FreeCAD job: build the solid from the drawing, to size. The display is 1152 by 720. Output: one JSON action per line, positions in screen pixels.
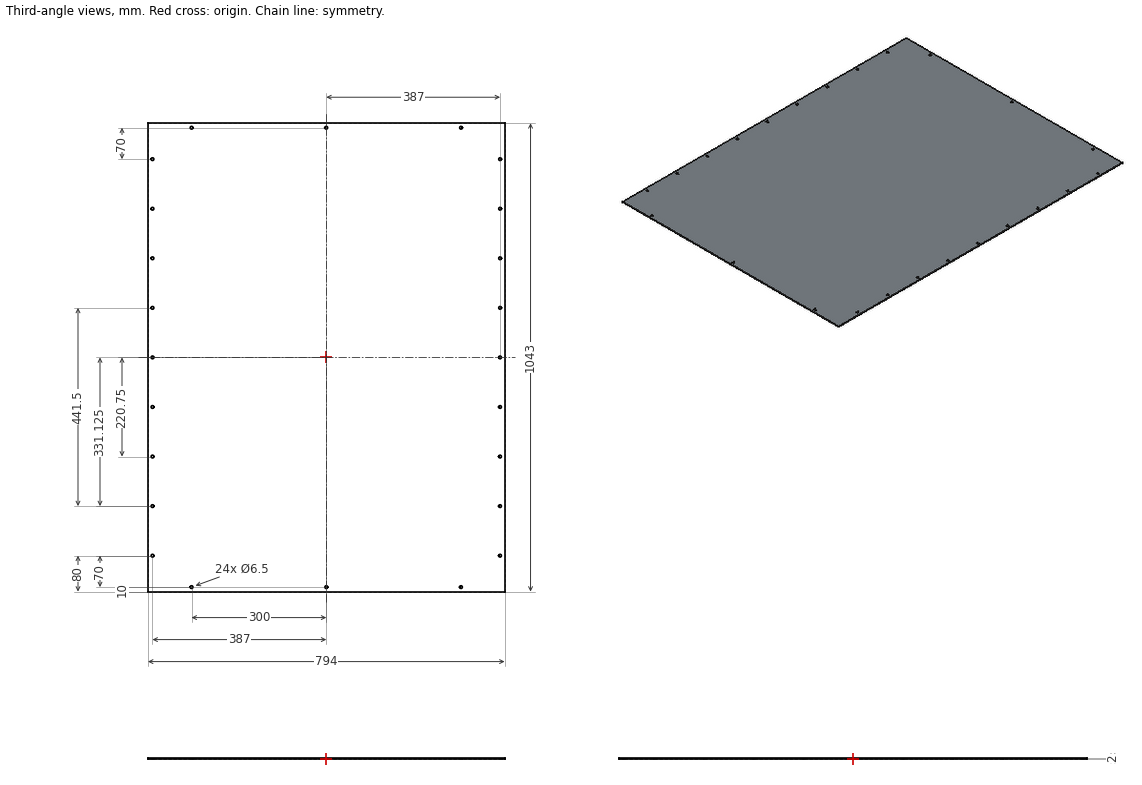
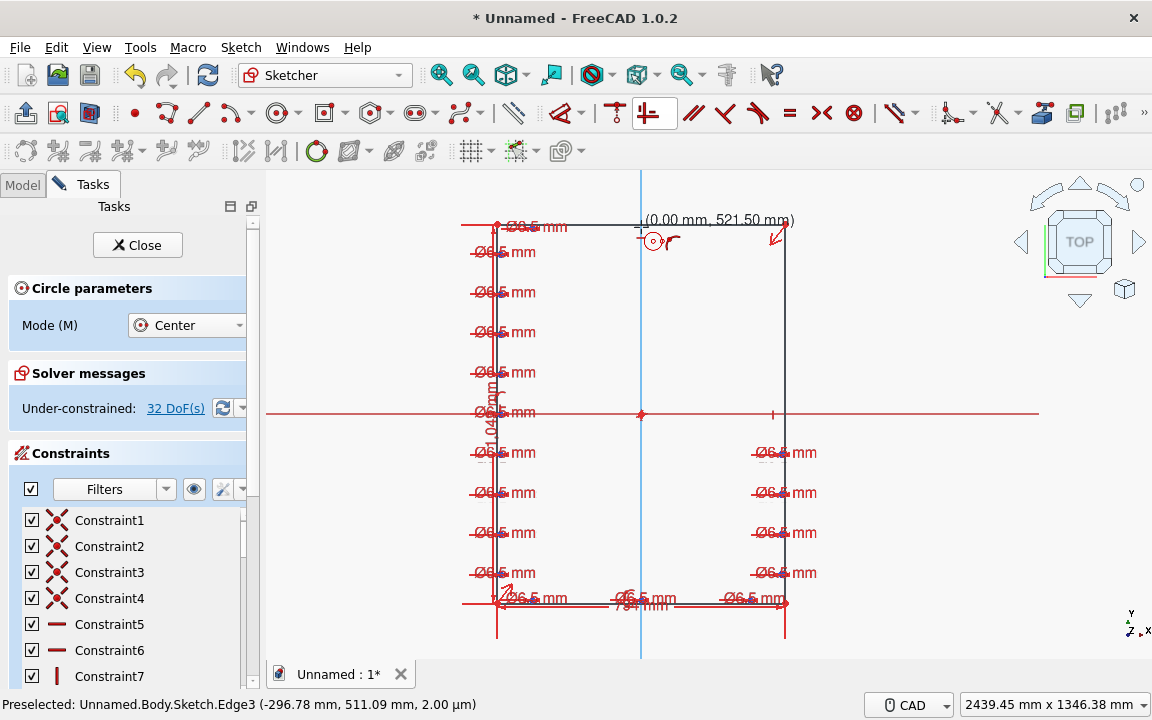
{"action": "scroll", "coordinate": [641, 229], "scroll_direction": "up", "scroll_amount": 8}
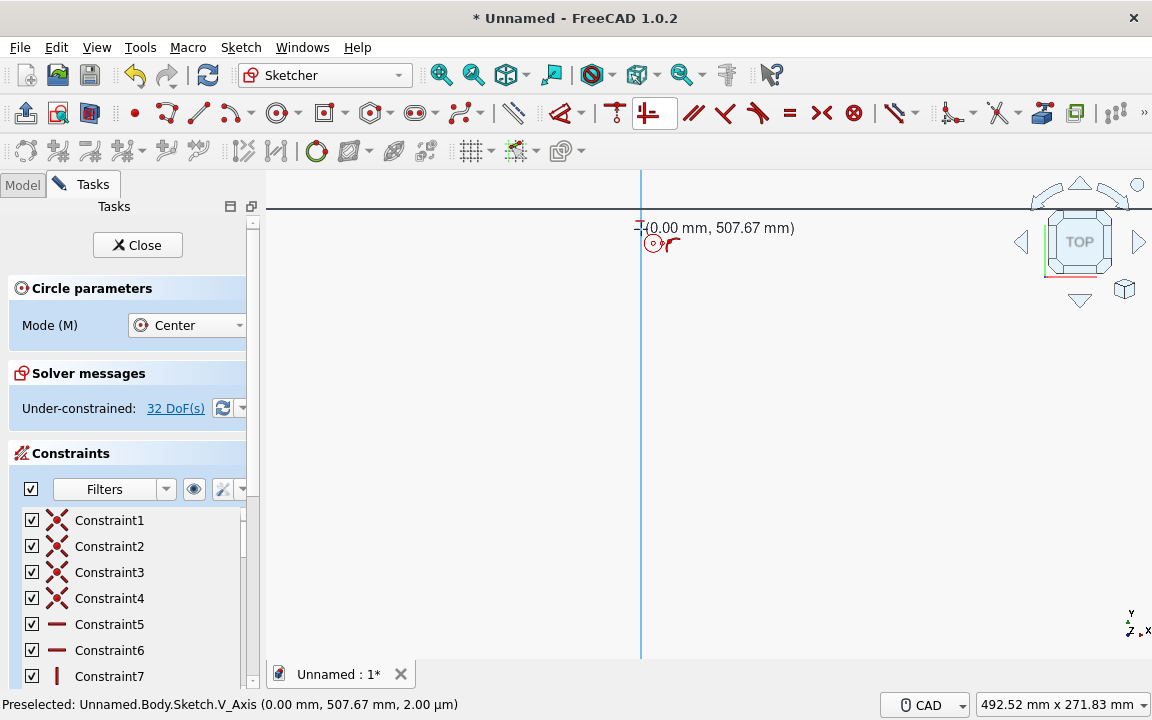
{"action": "left_click", "coordinate": [641, 227]}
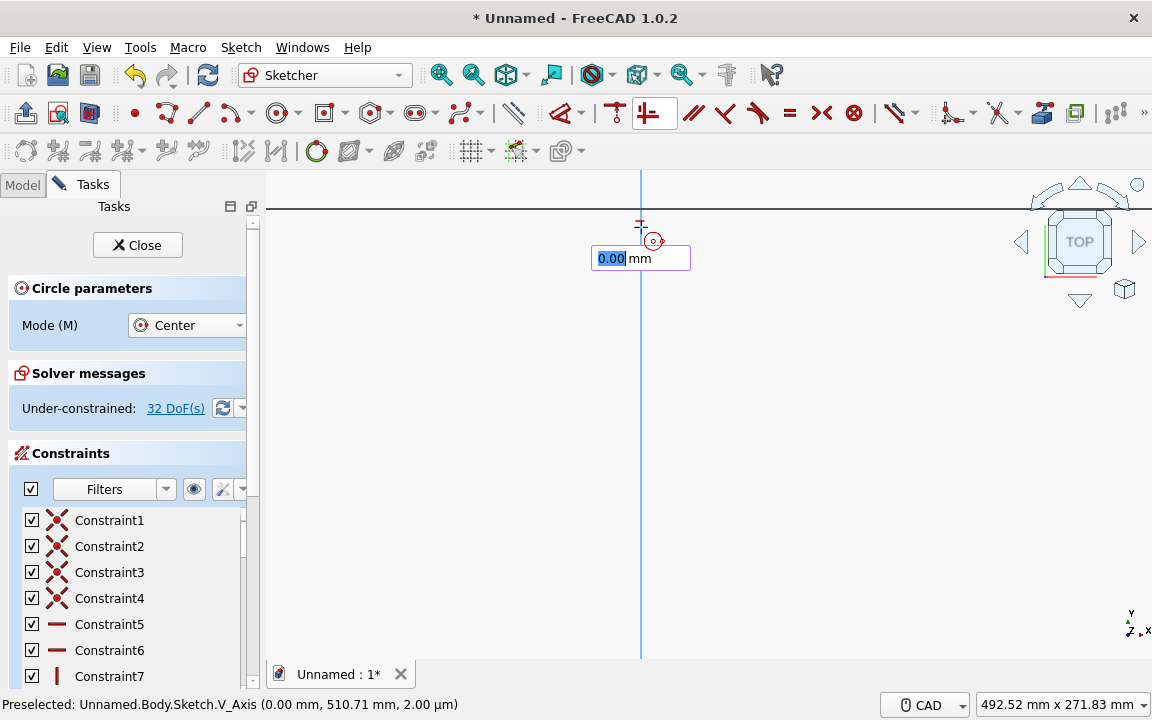
{"action": "scroll", "coordinate": [646, 225], "scroll_direction": "up", "scroll_amount": 6}
{"action": "mouse_move", "coordinate": [646, 223]}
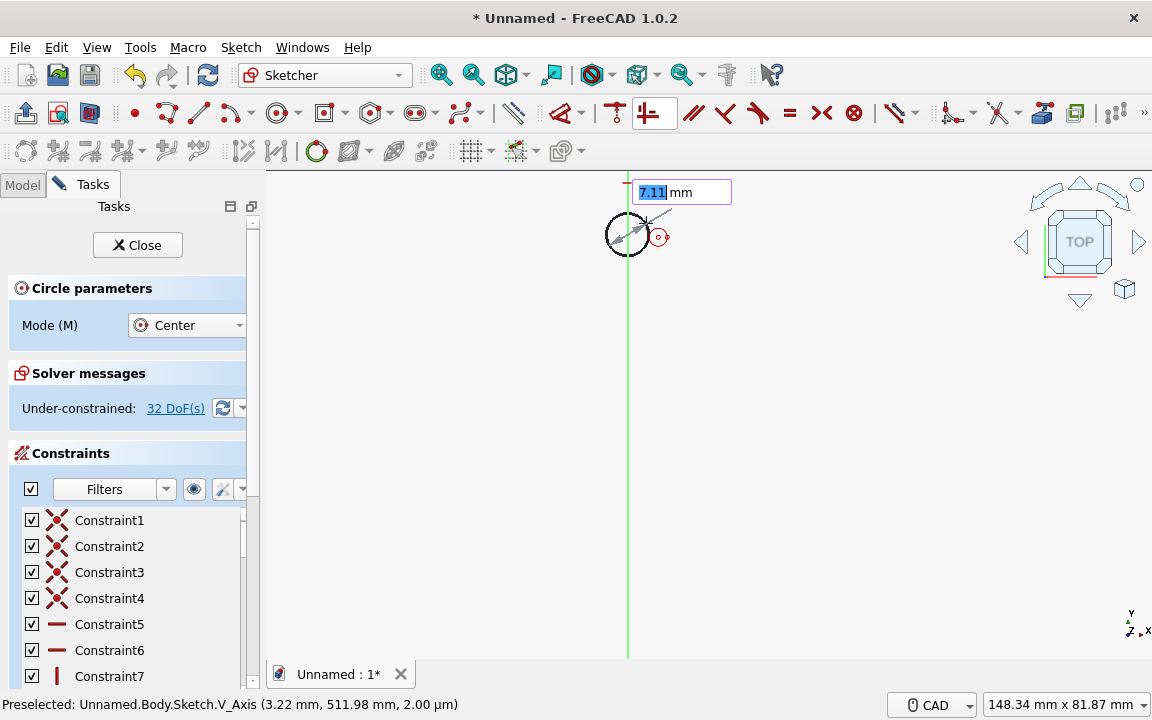
{"action": "type", "text": "6.5"}
{"action": "key", "text": "Return"}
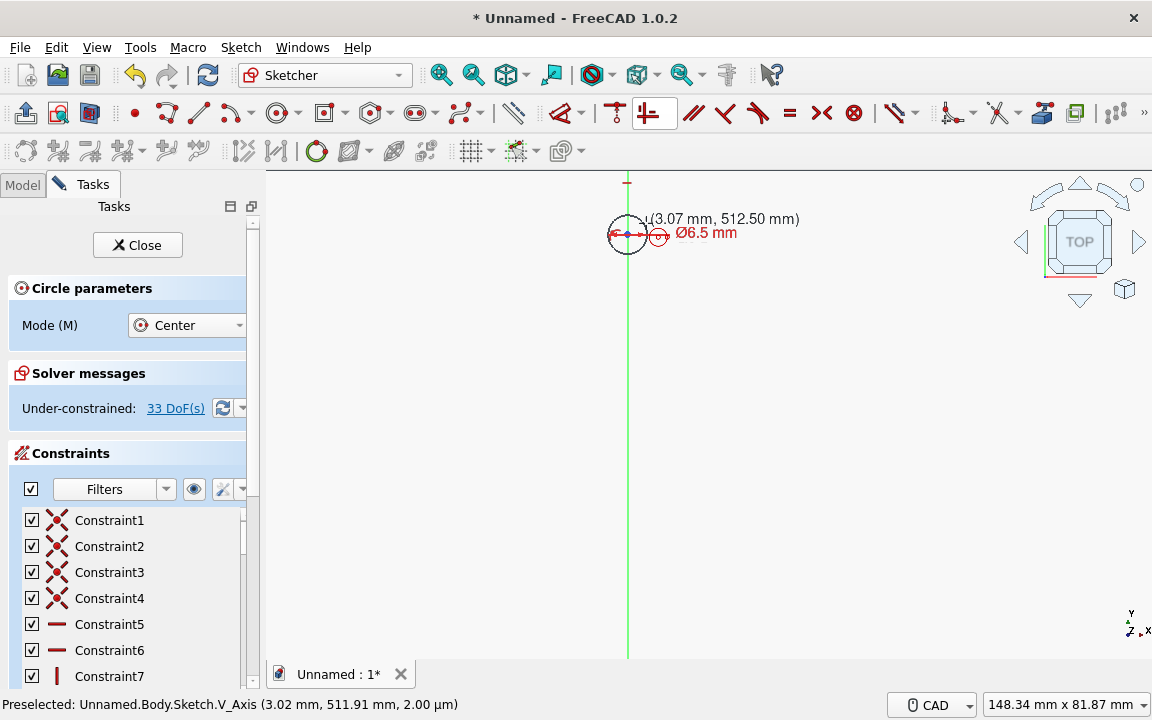
{"action": "scroll", "coordinate": [641, 264], "scroll_direction": "down", "scroll_amount": 15}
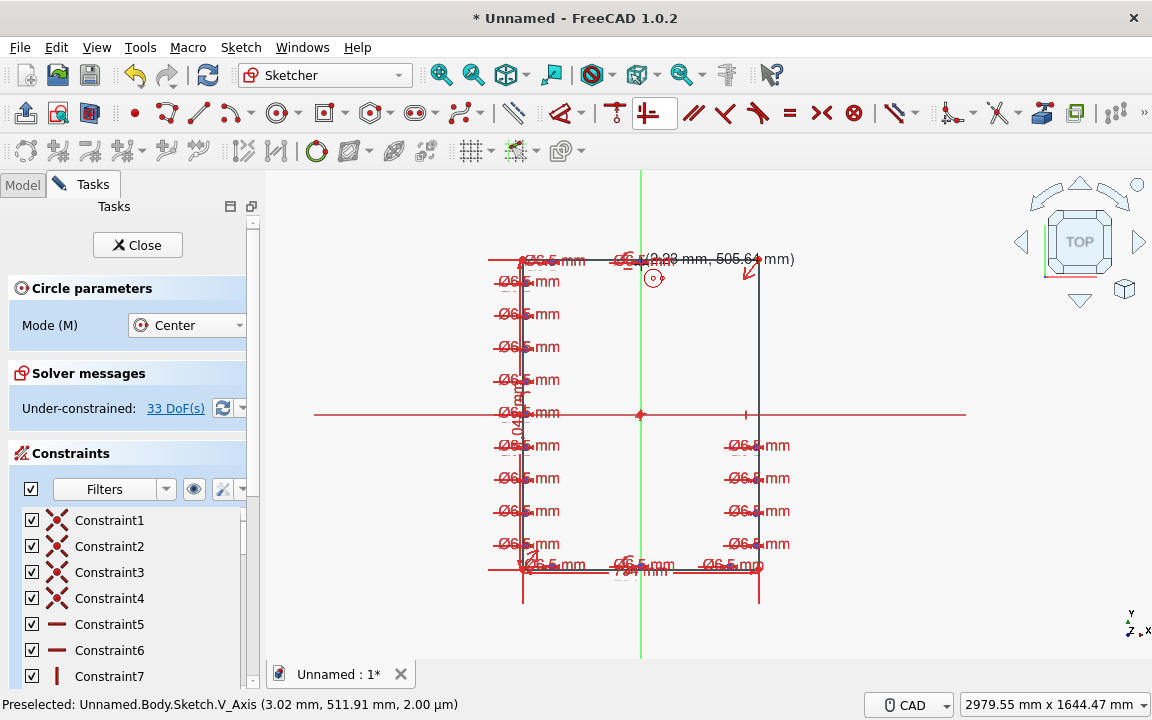
{"action": "scroll", "coordinate": [756, 415], "scroll_direction": "up", "scroll_amount": 16}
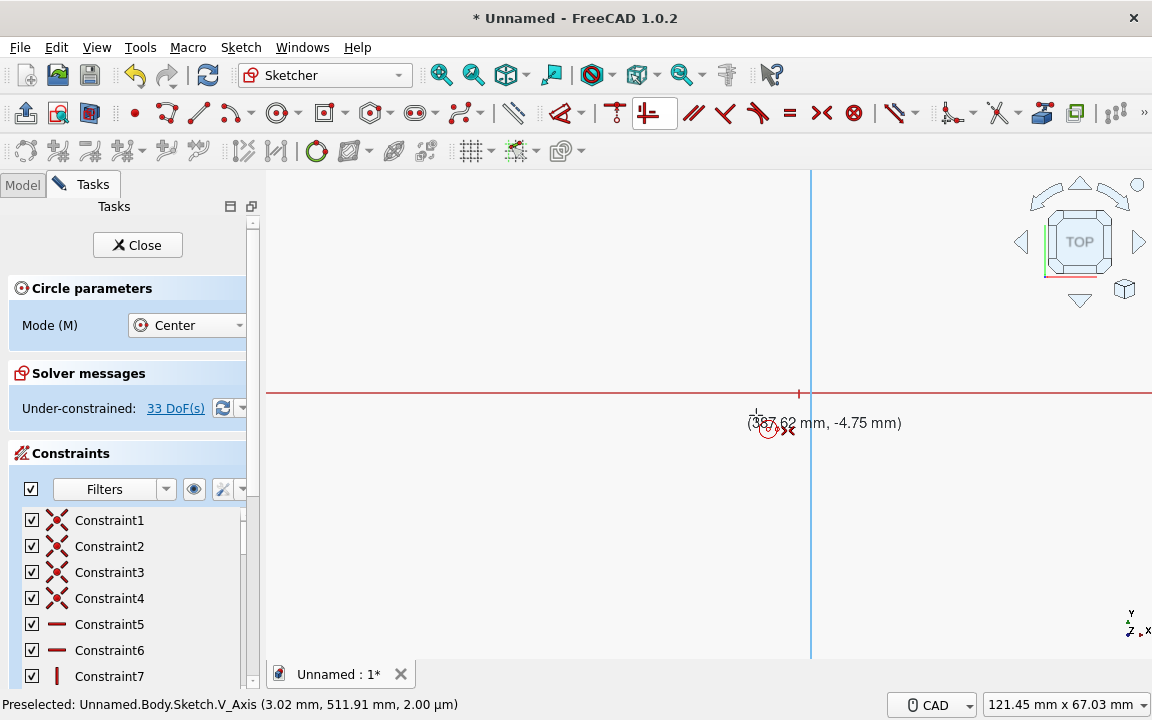
{"action": "scroll", "coordinate": [783, 416], "scroll_direction": "down", "scroll_amount": 15}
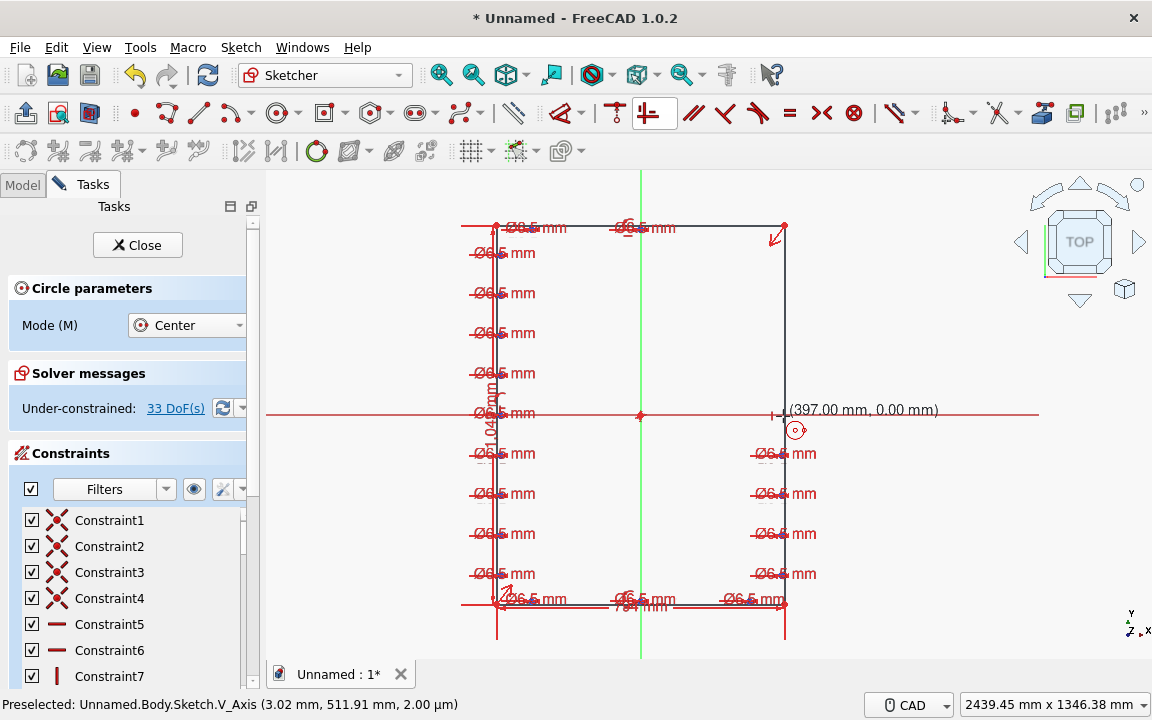
{"action": "scroll", "coordinate": [781, 415], "scroll_direction": "up", "scroll_amount": 8}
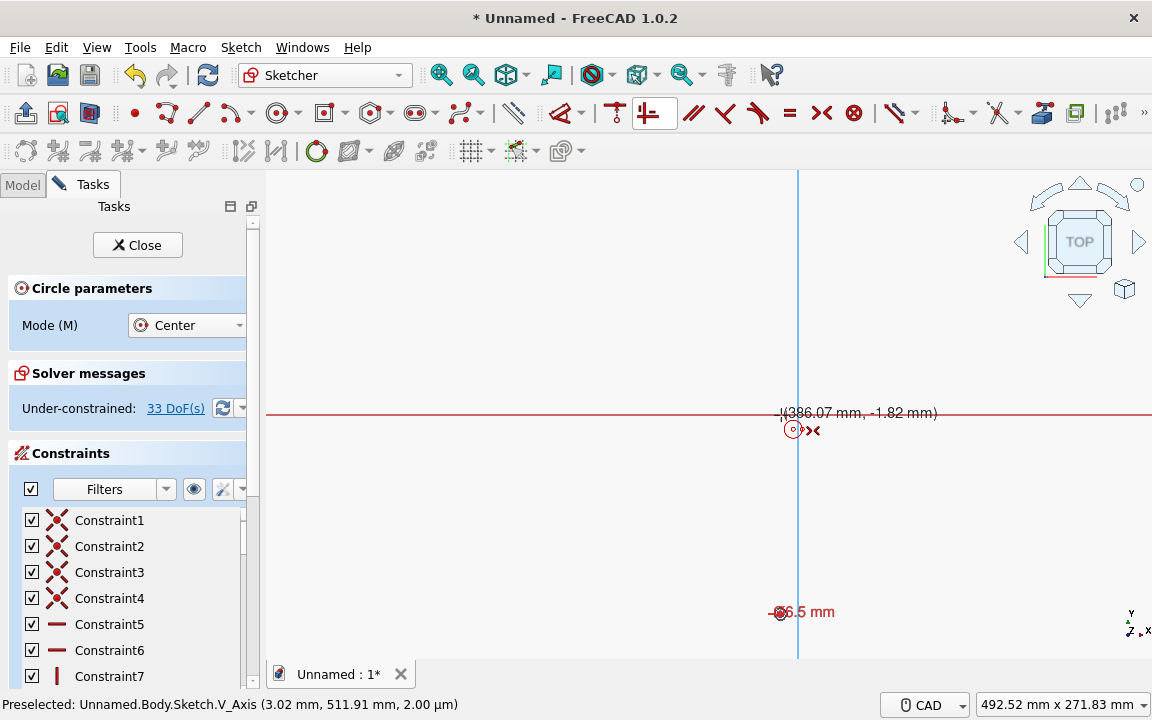
{"action": "left_click", "coordinate": [780, 415]}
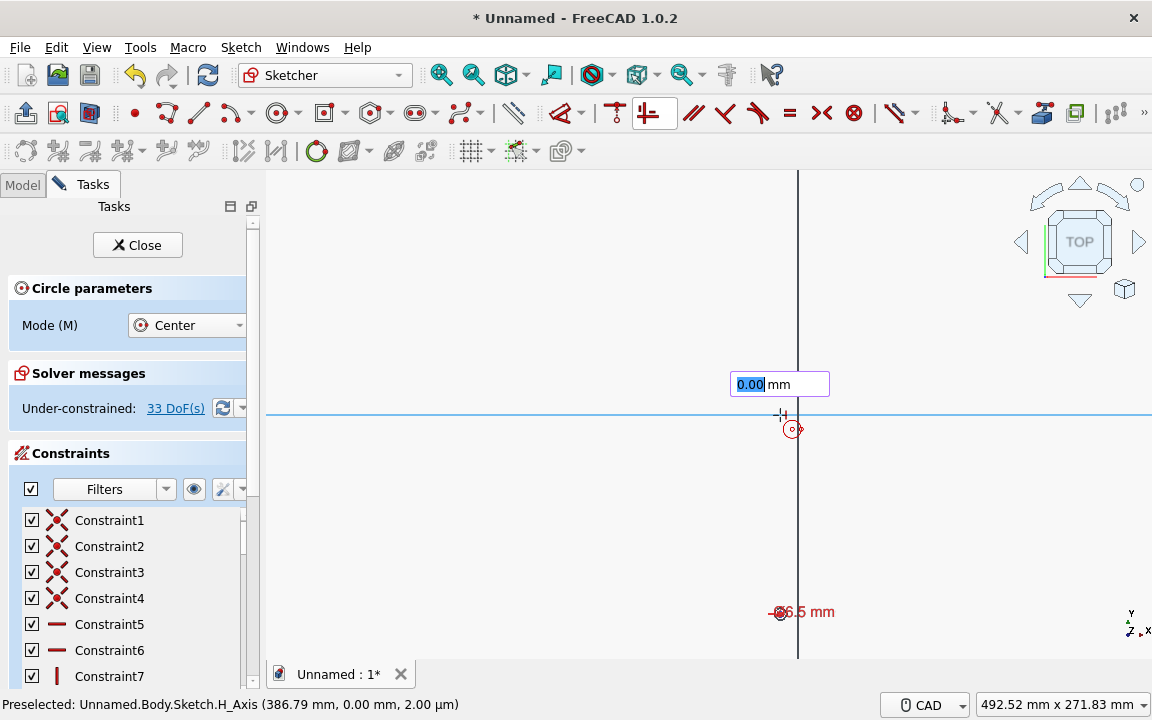
{"action": "scroll", "coordinate": [778, 420], "scroll_direction": "up", "scroll_amount": 6}
{"action": "mouse_move", "coordinate": [778, 419]}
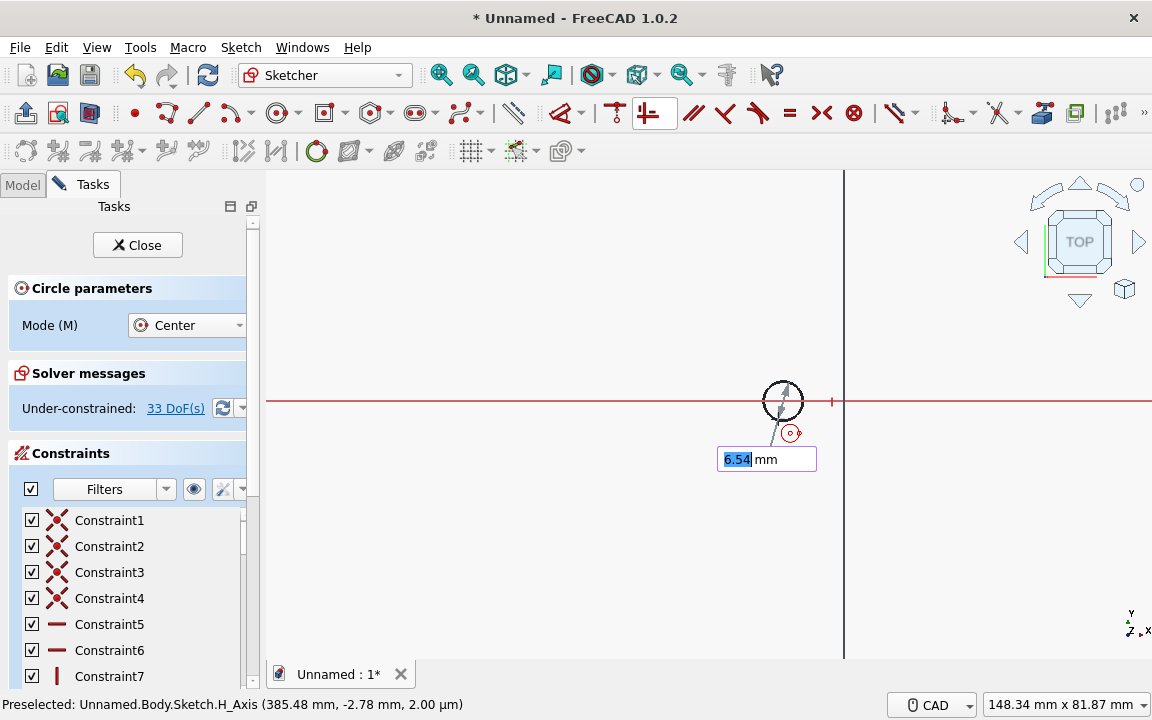
{"action": "type", "text": "6.5"}
{"action": "key", "text": "Return"}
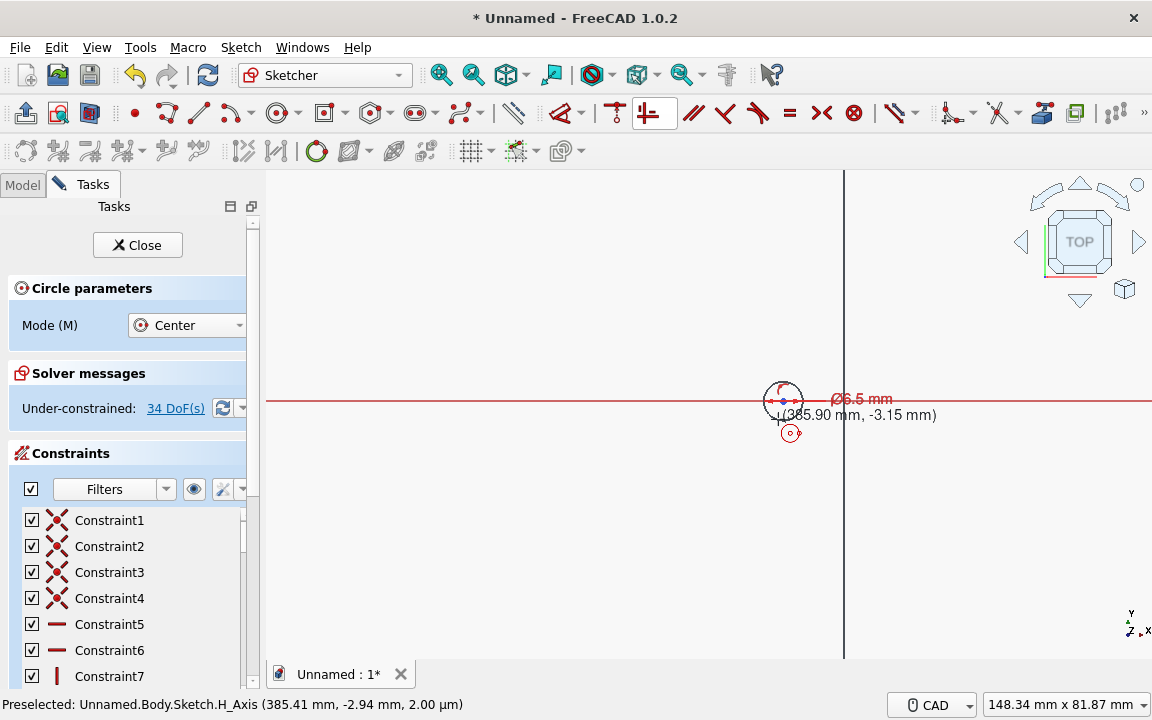
{"action": "scroll", "coordinate": [754, 415], "scroll_direction": "down", "scroll_amount": 15}